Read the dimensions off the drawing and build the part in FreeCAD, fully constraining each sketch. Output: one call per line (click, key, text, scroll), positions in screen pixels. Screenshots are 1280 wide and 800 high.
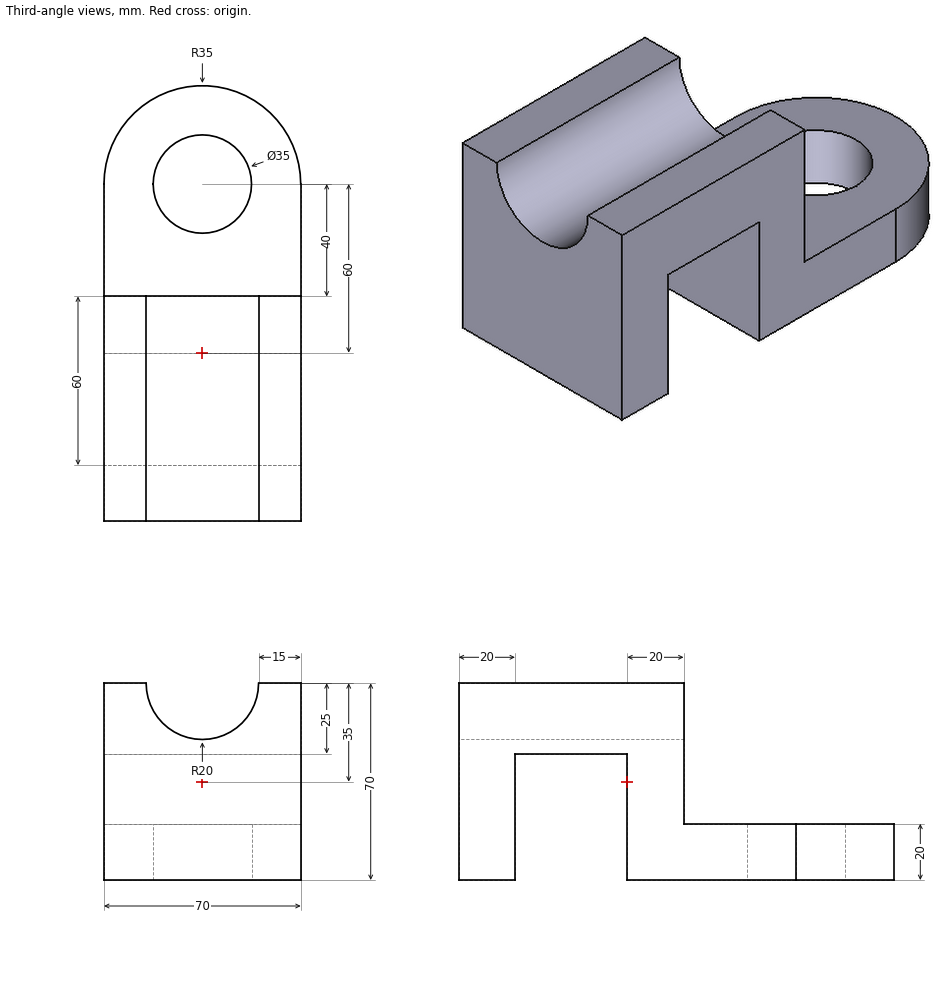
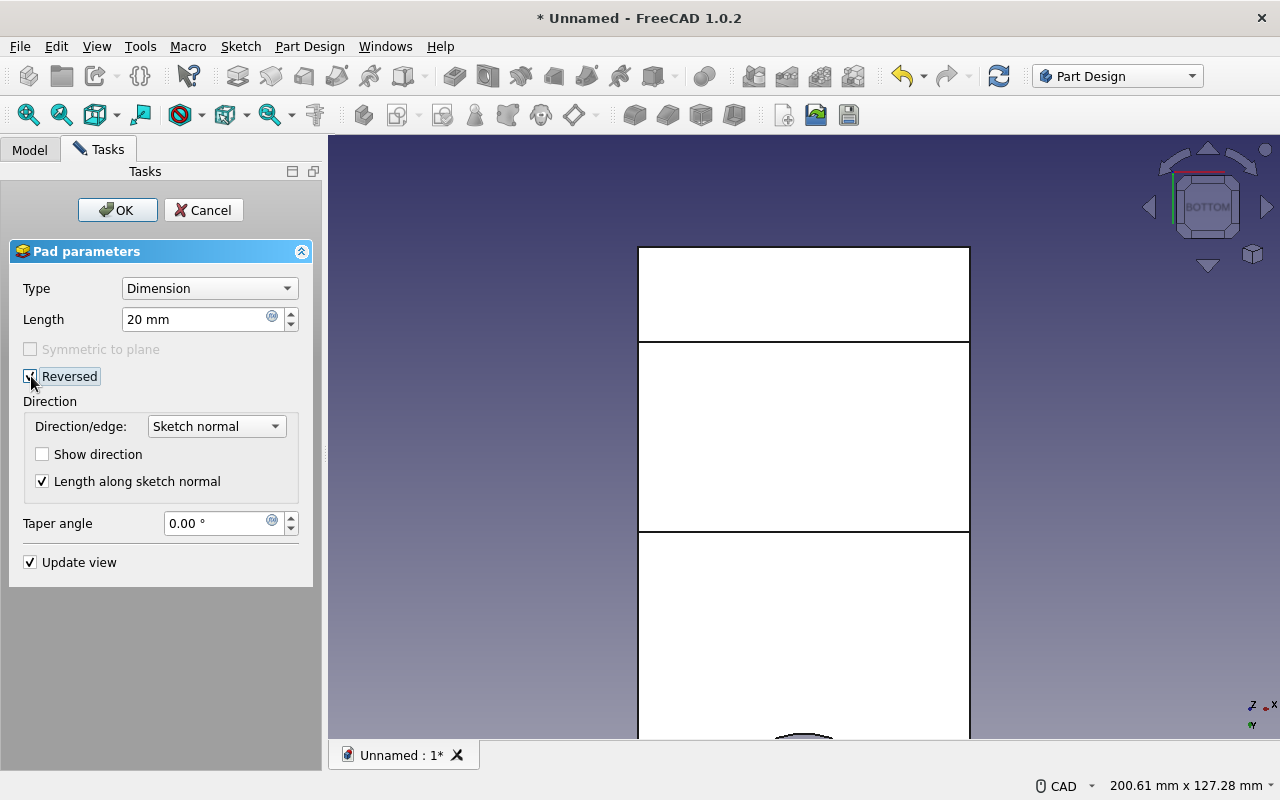
click(118, 210)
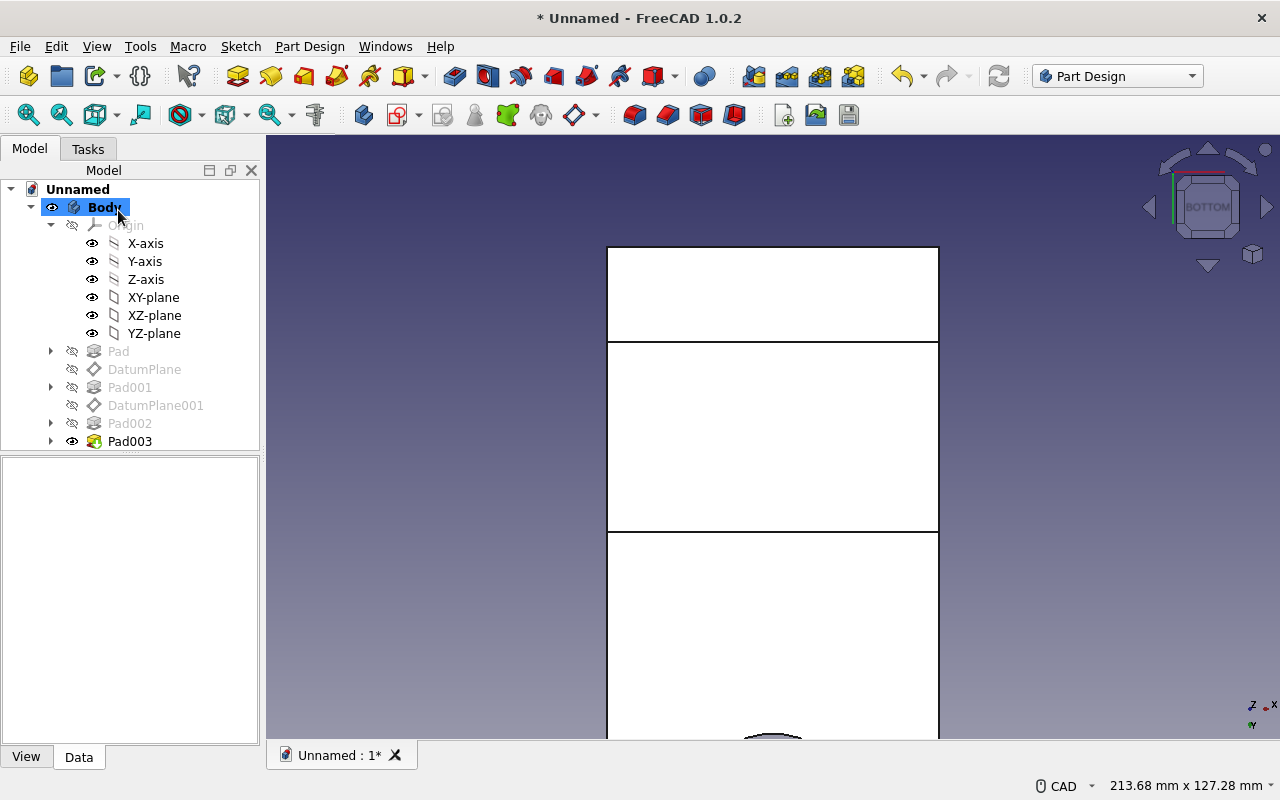
key(0)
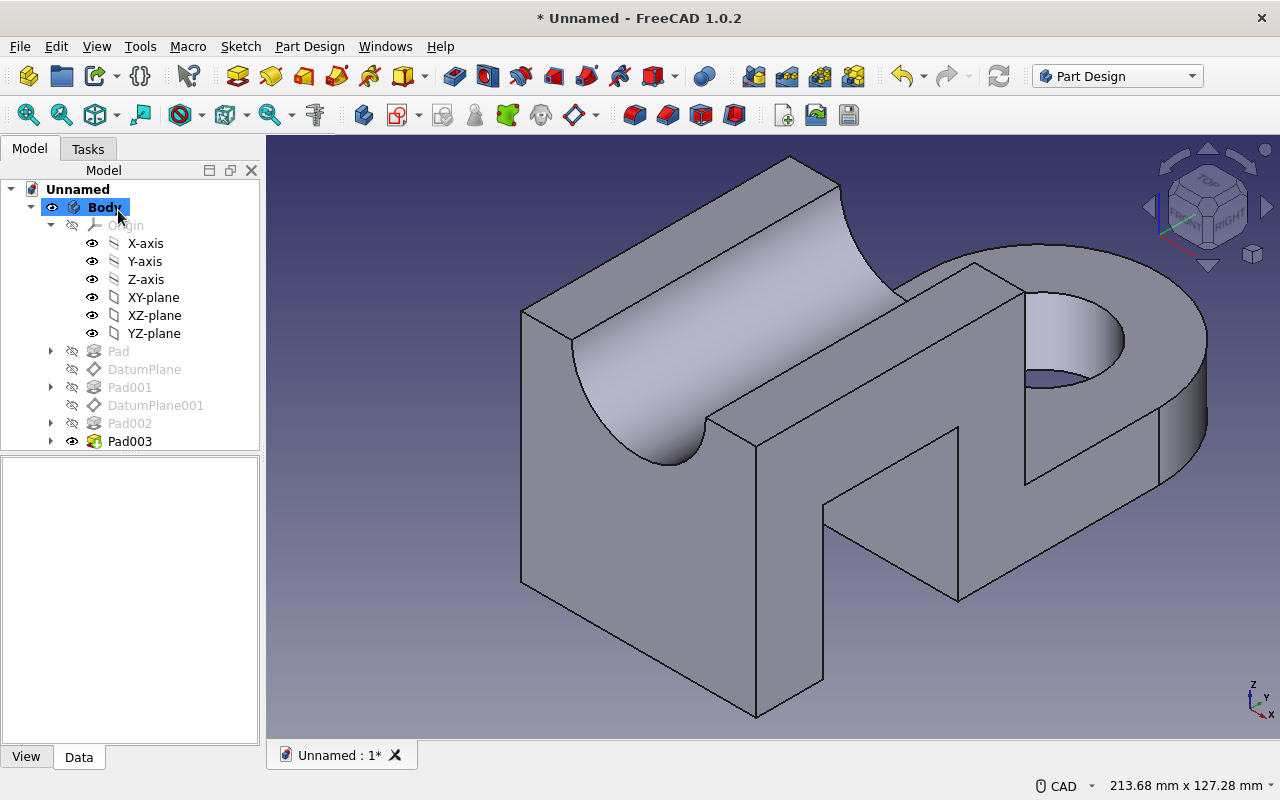
click(29, 116)